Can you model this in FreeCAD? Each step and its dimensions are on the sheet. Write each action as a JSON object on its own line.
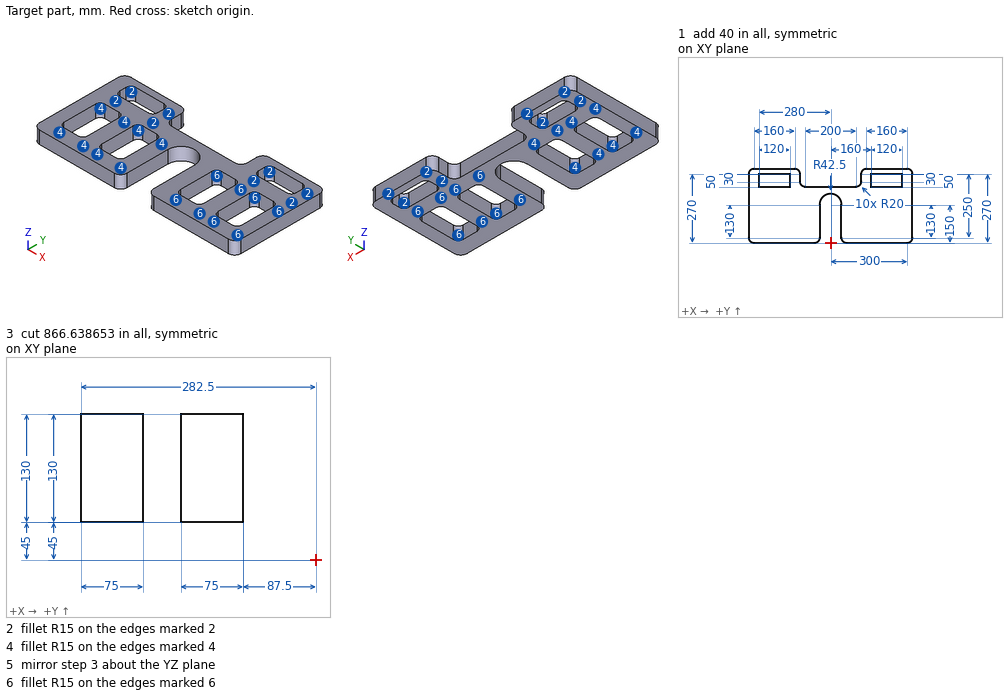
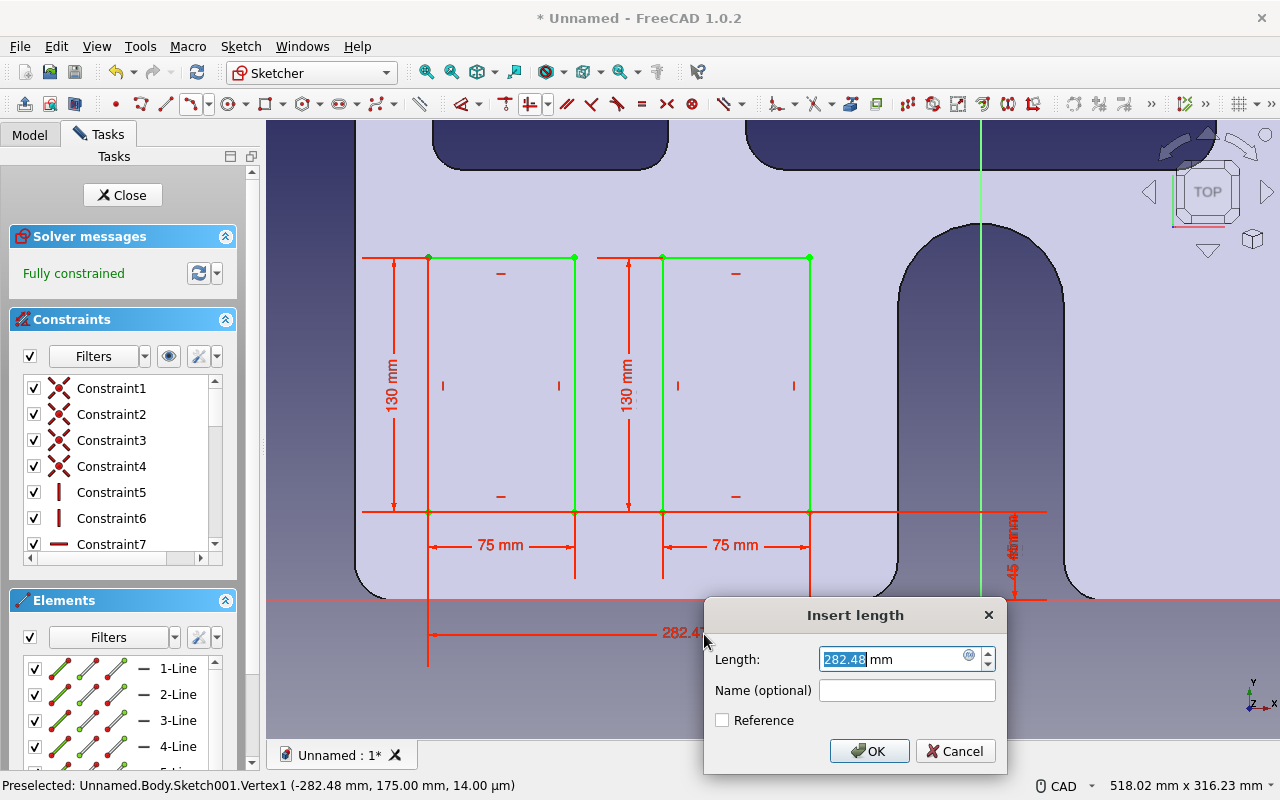
{"action": "type", "text": "282.5"}
{"action": "key", "text": "Return"}
{"action": "key", "text": "Escape"}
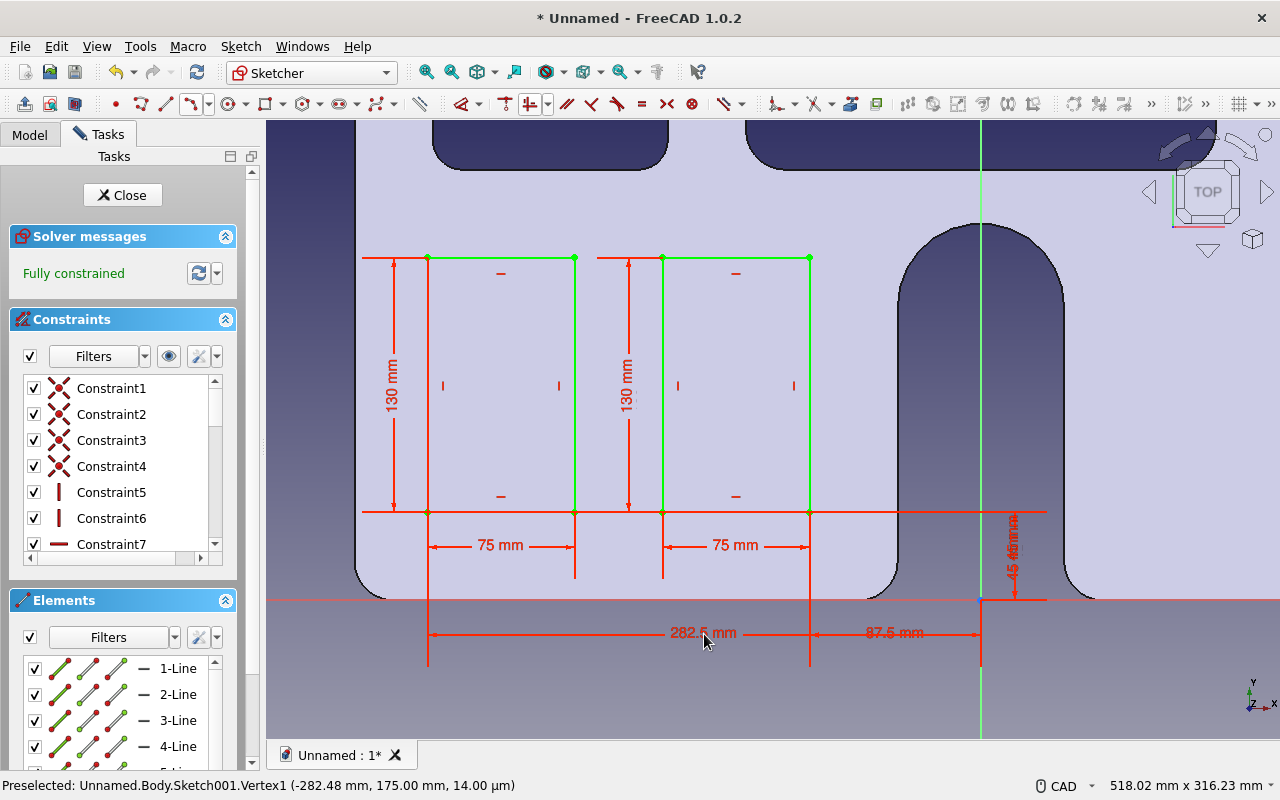
{"action": "left_click", "coordinate": [123, 195]}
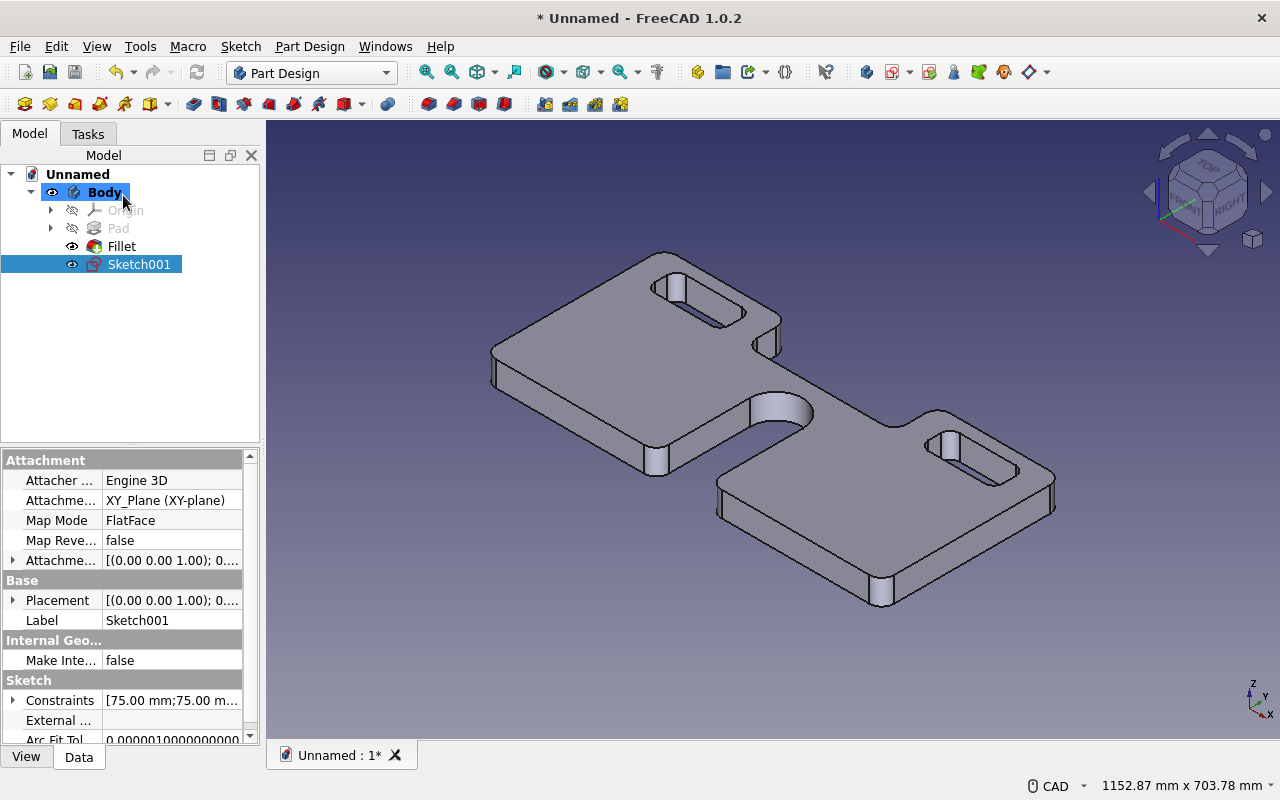
{"action": "left_click", "coordinate": [194, 104]}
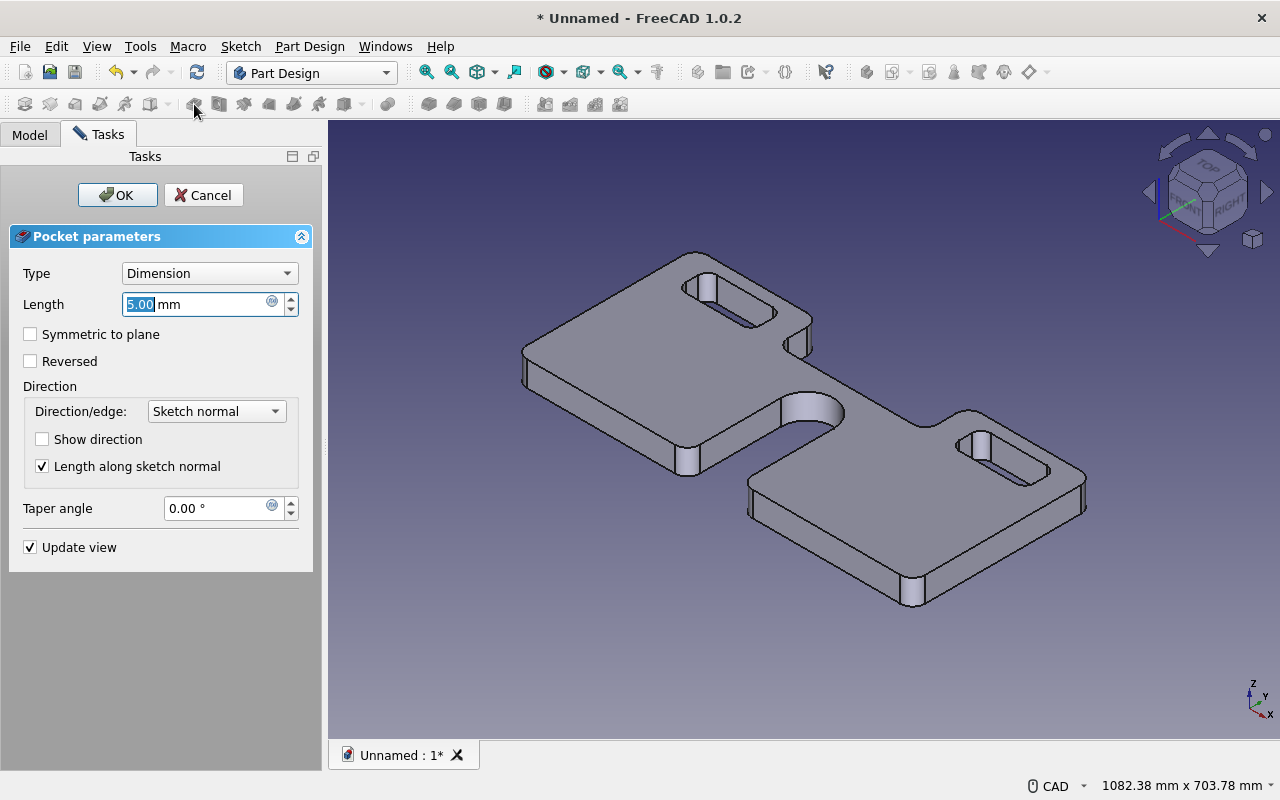
{"action": "type", "text": "866.638653"}
{"action": "key", "text": "Tab"}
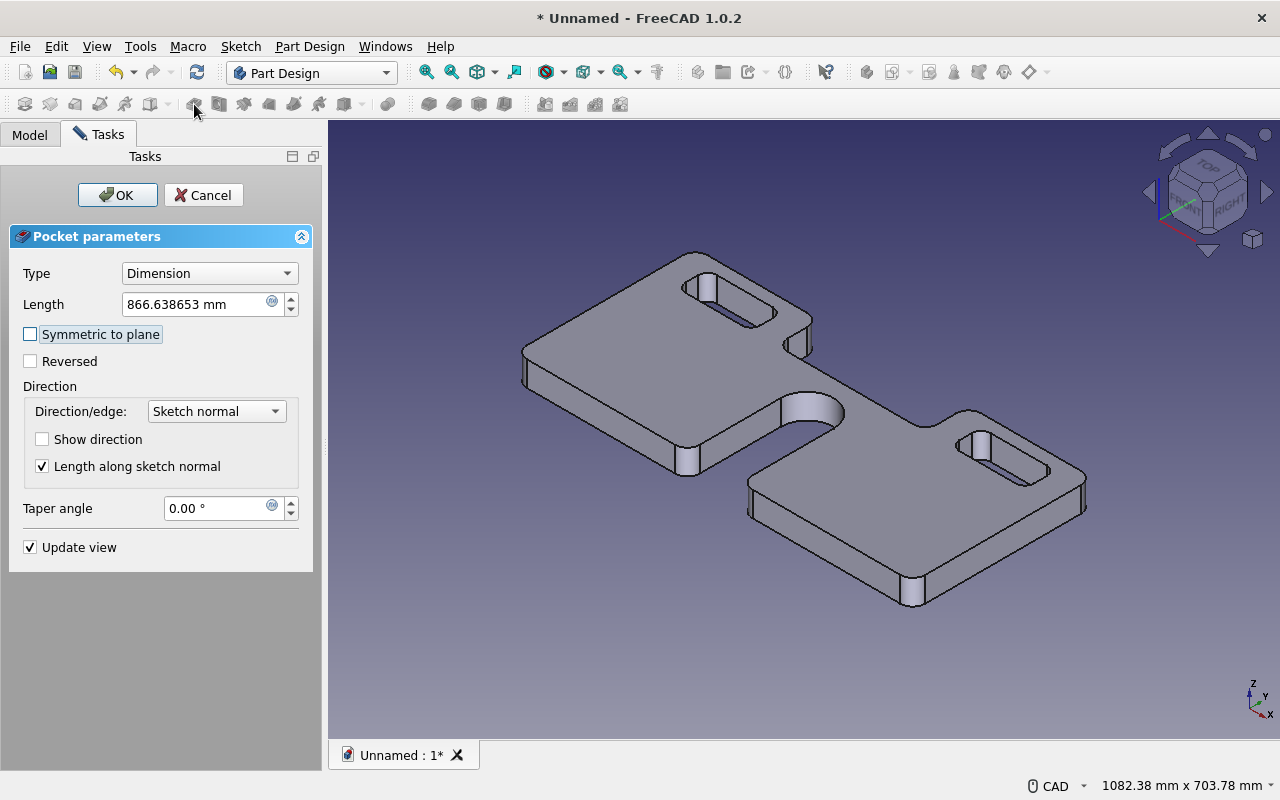
{"action": "left_click", "coordinate": [31, 334]}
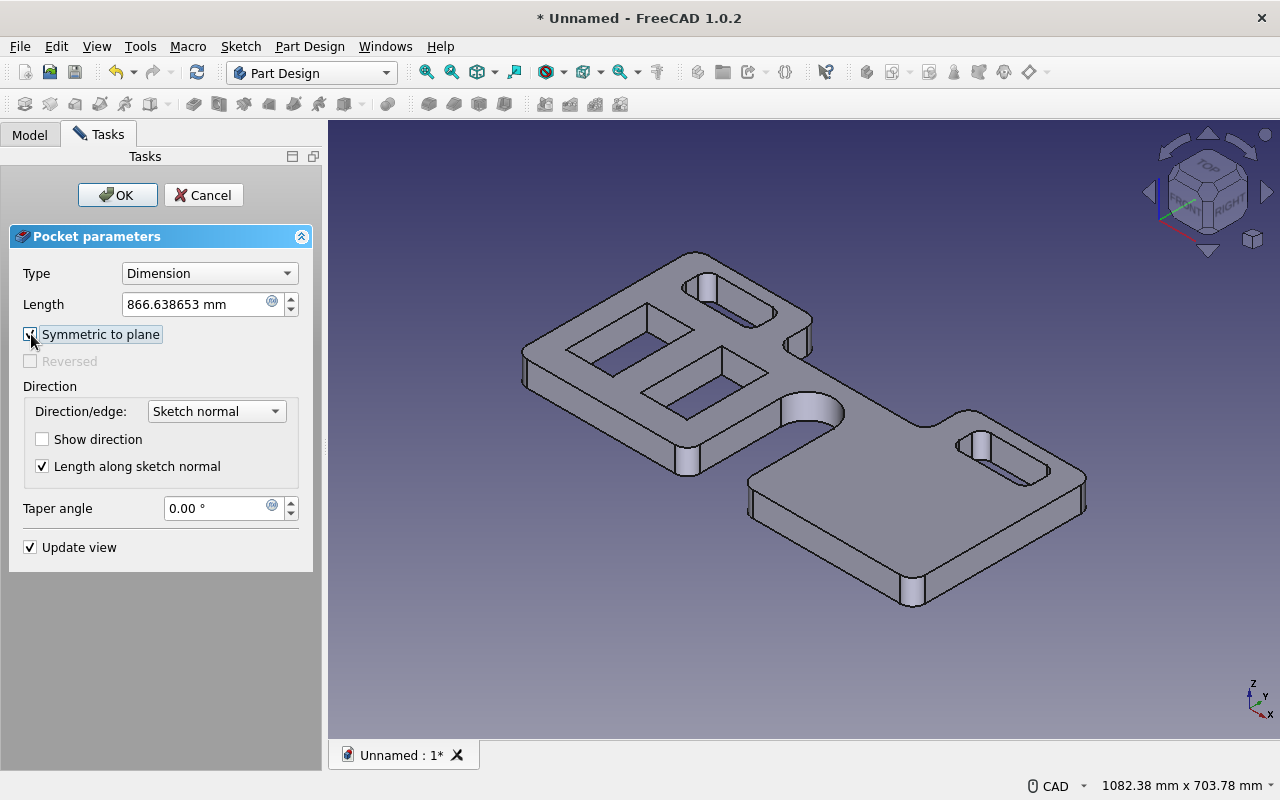
{"action": "left_click", "coordinate": [118, 195]}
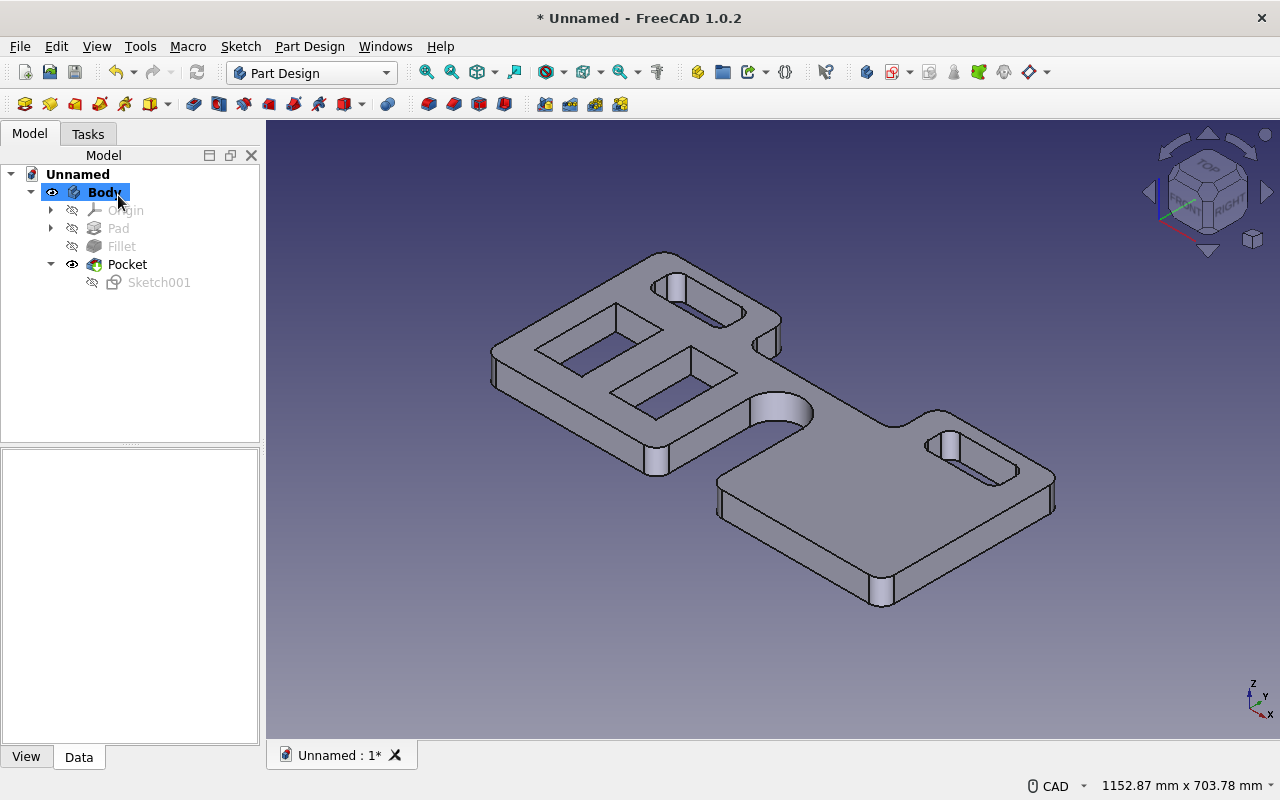
{"action": "key", "text": "2"}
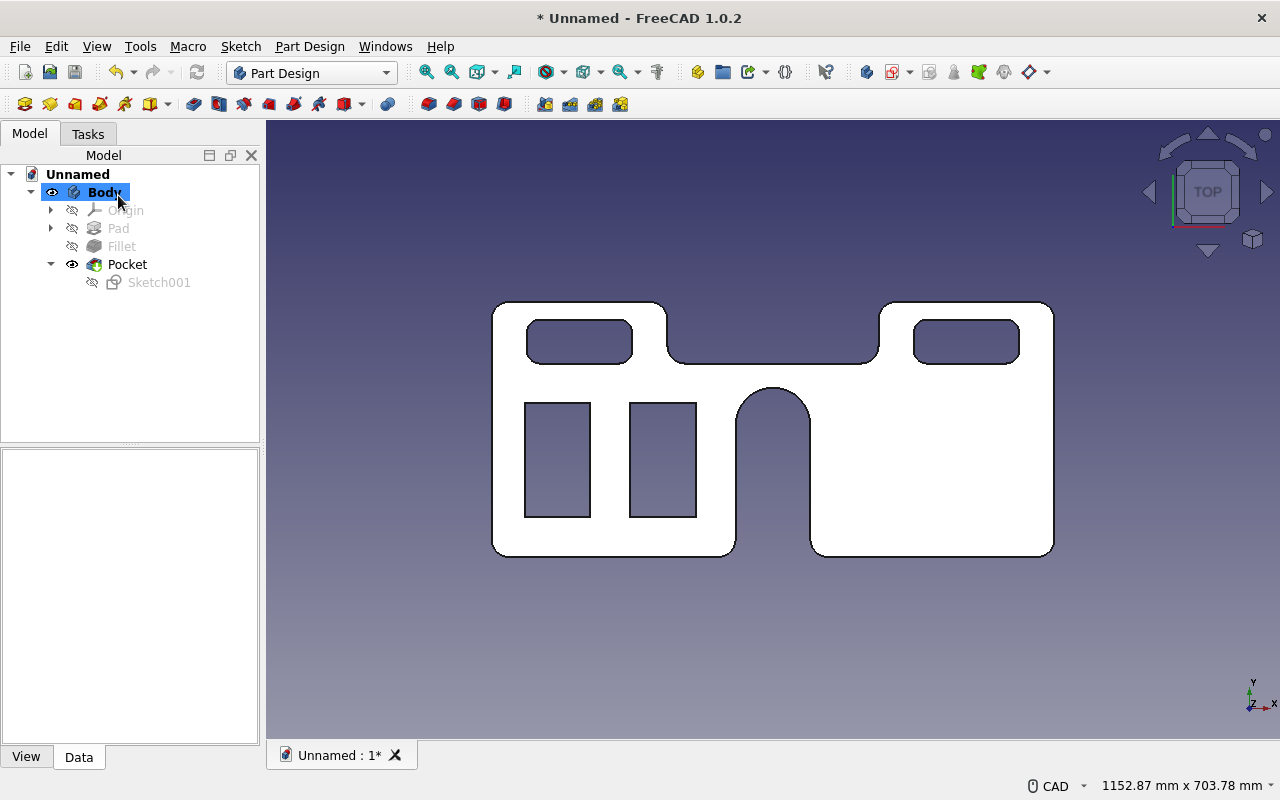
{"action": "key", "text": "0"}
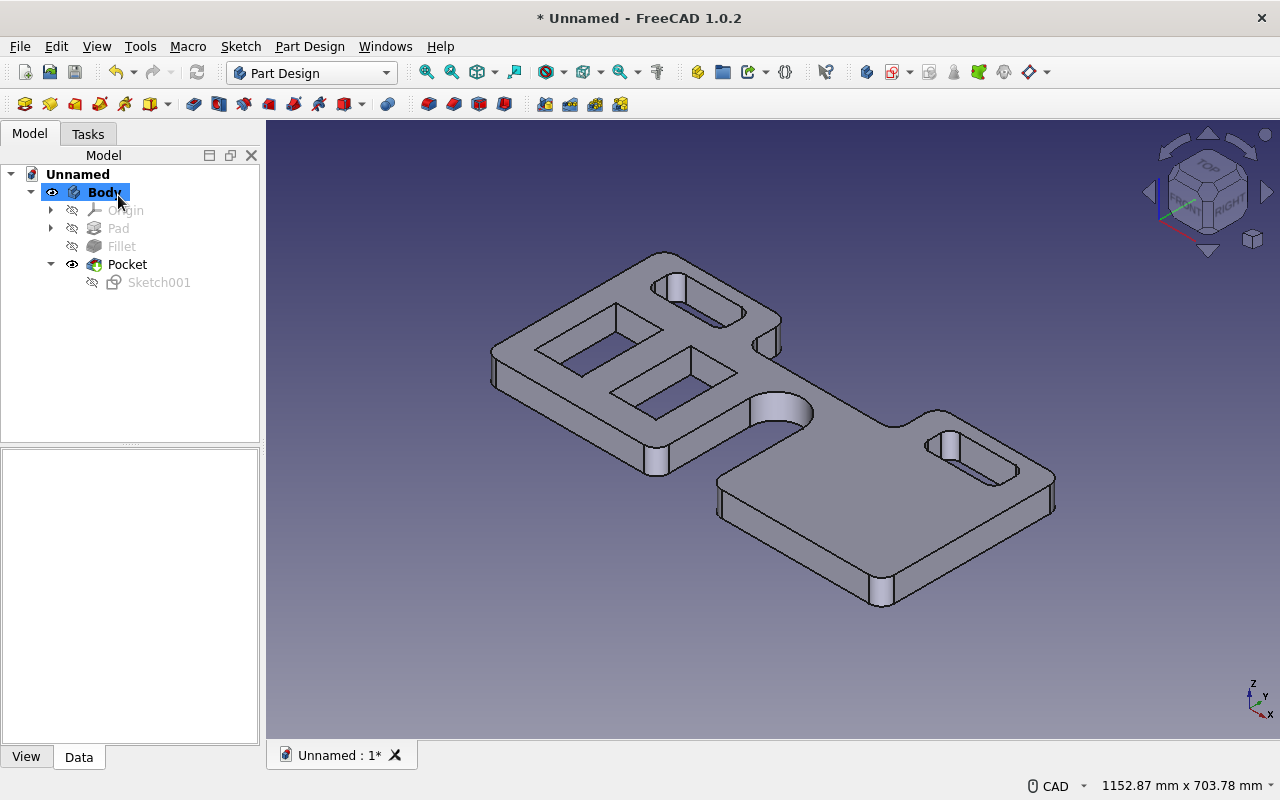
{"action": "key", "text": "1"}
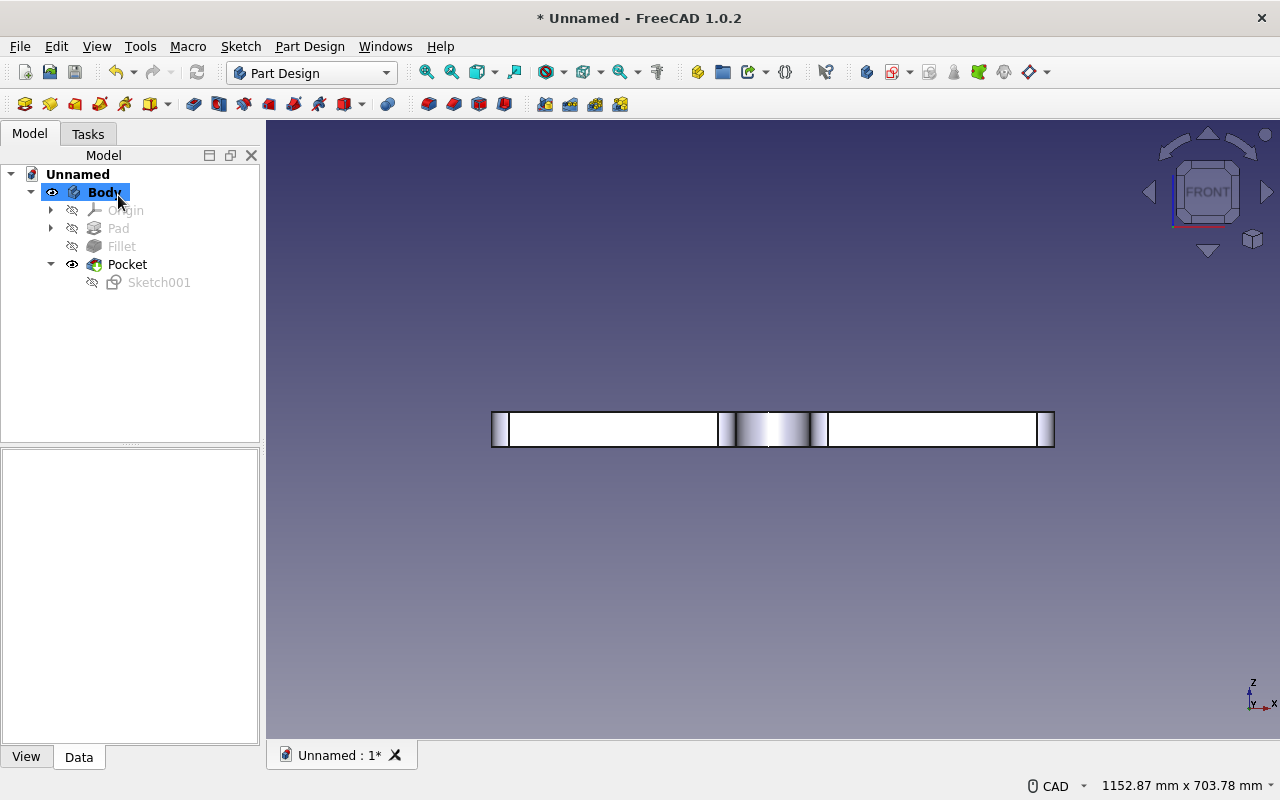
{"action": "key", "text": "3"}